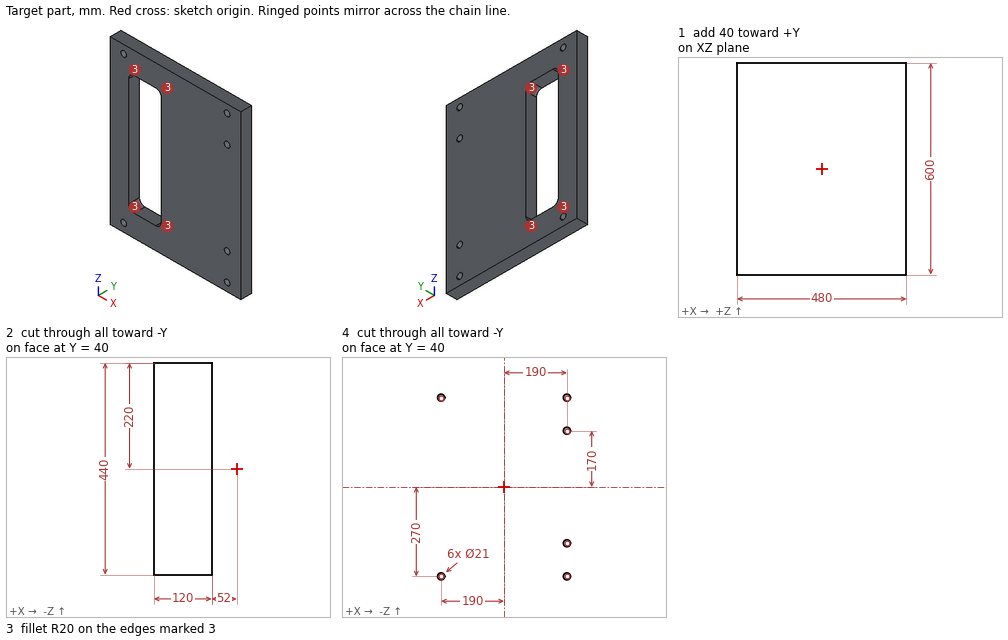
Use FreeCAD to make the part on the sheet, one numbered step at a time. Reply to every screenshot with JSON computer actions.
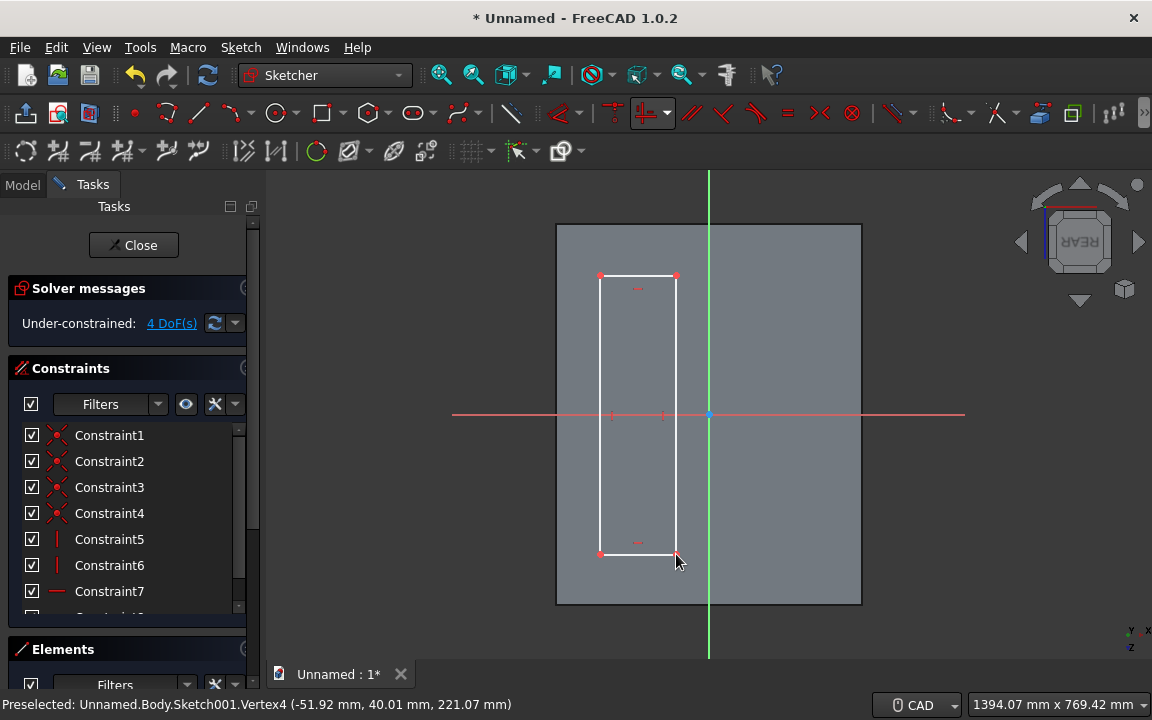
{"action": "left_click", "coordinate": [600, 360]}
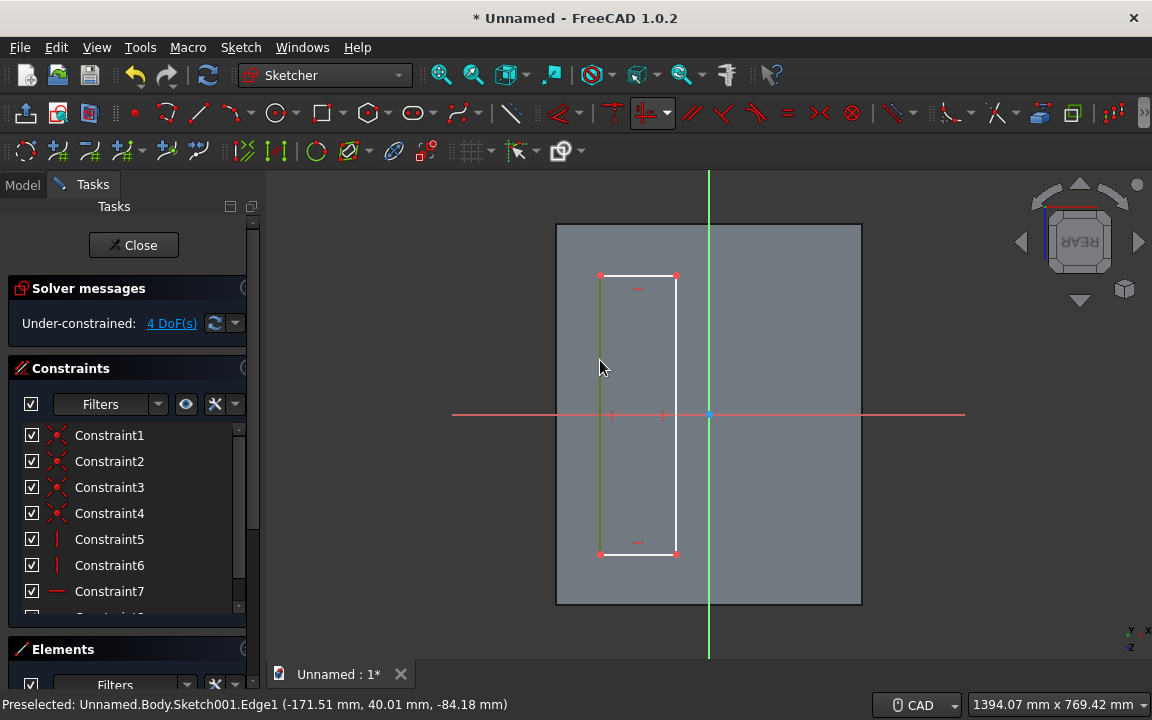
{"action": "left_click", "coordinate": [582, 114]}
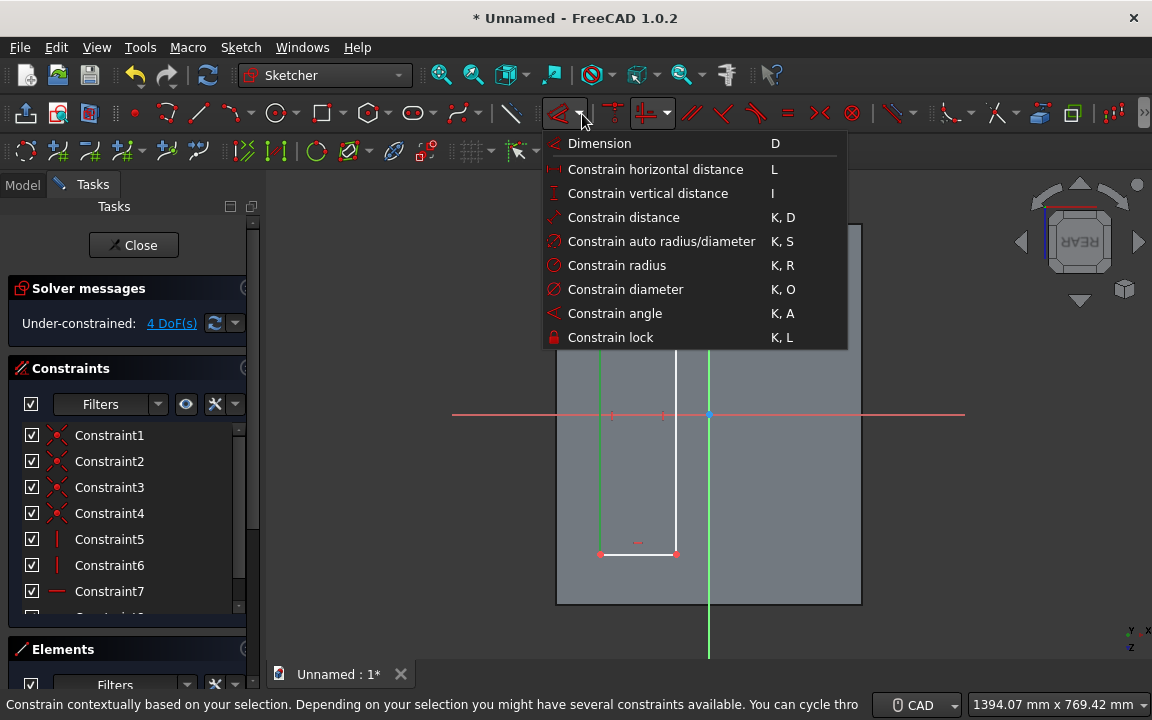
{"action": "left_click", "coordinate": [695, 193]}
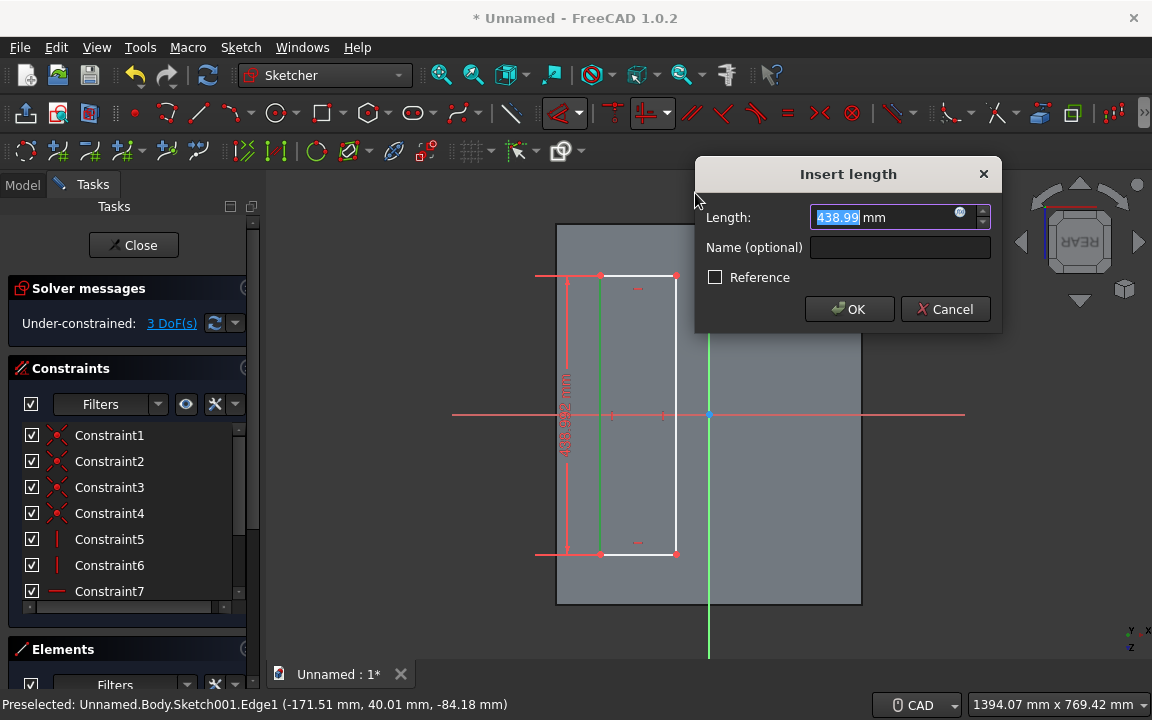
{"action": "type", "text": "440"}
{"action": "key", "text": "Return"}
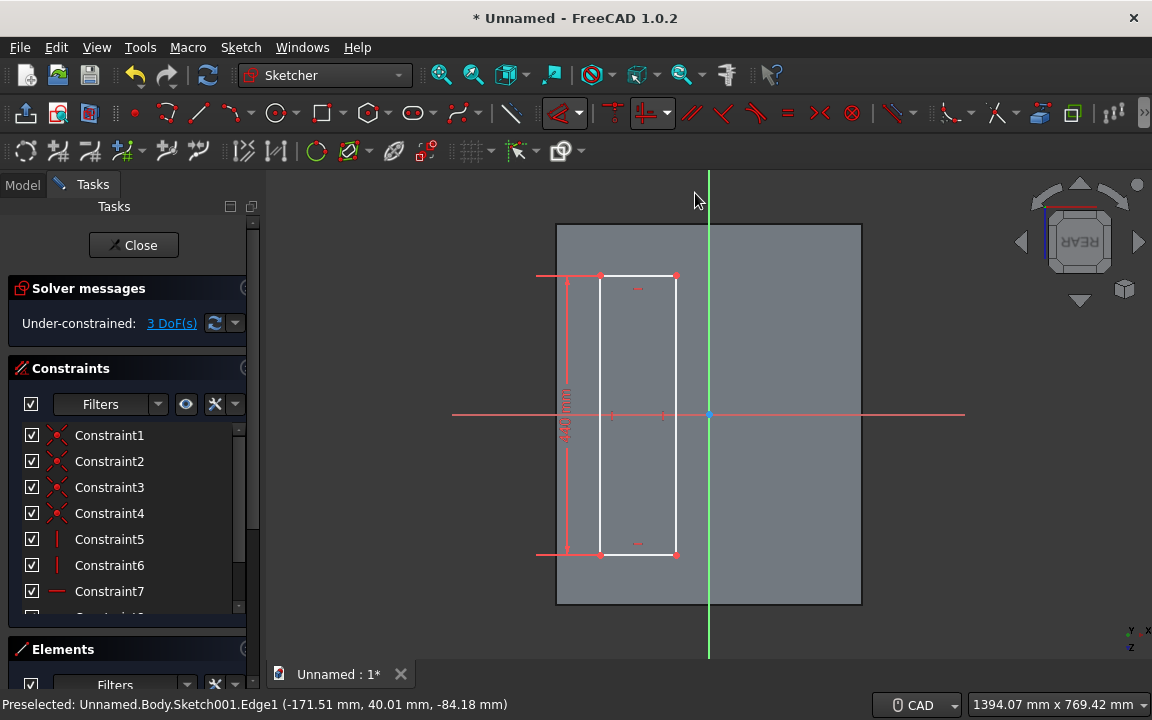
{"action": "left_click", "coordinate": [623, 555]}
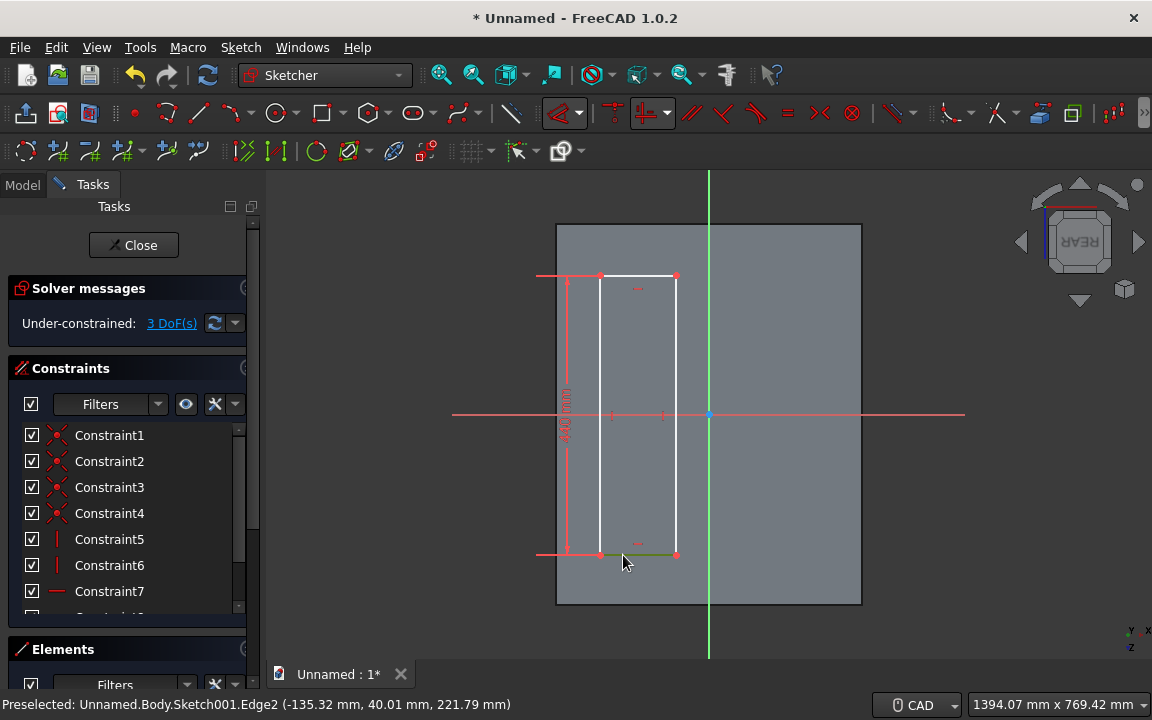
{"action": "key", "text": "l"}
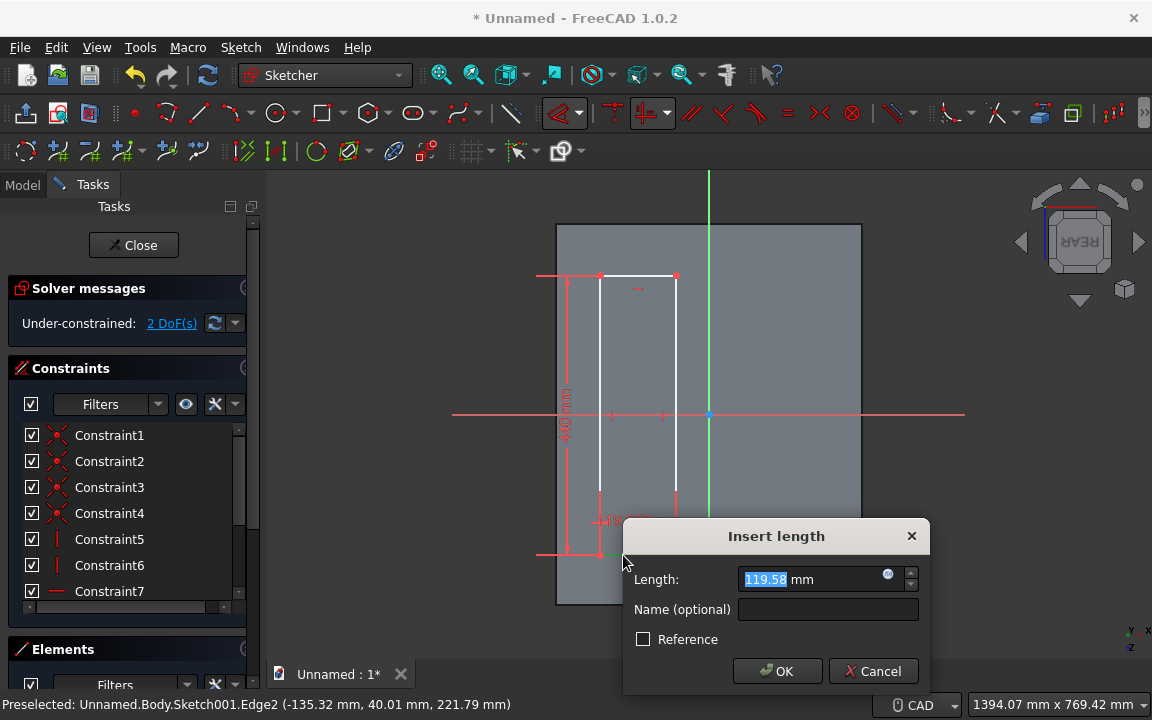
{"action": "type", "text": "120"}
{"action": "key", "text": "Return"}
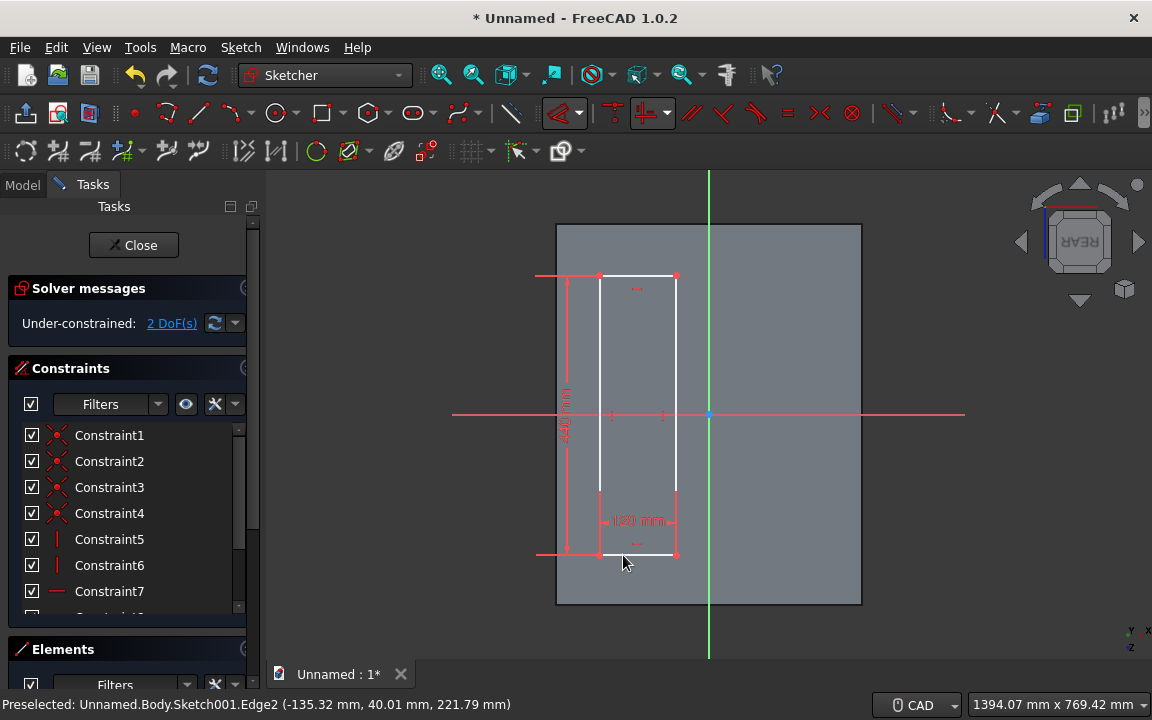
{"action": "left_click", "coordinate": [676, 555]}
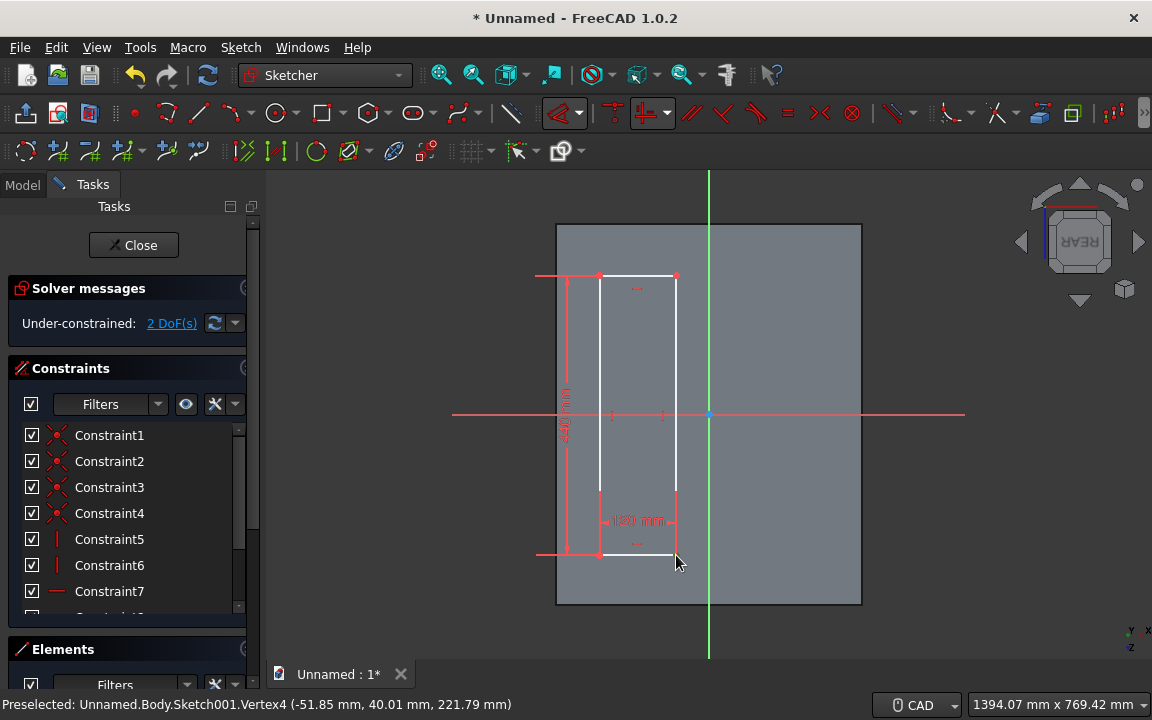
{"action": "left_click", "coordinate": [582, 114]}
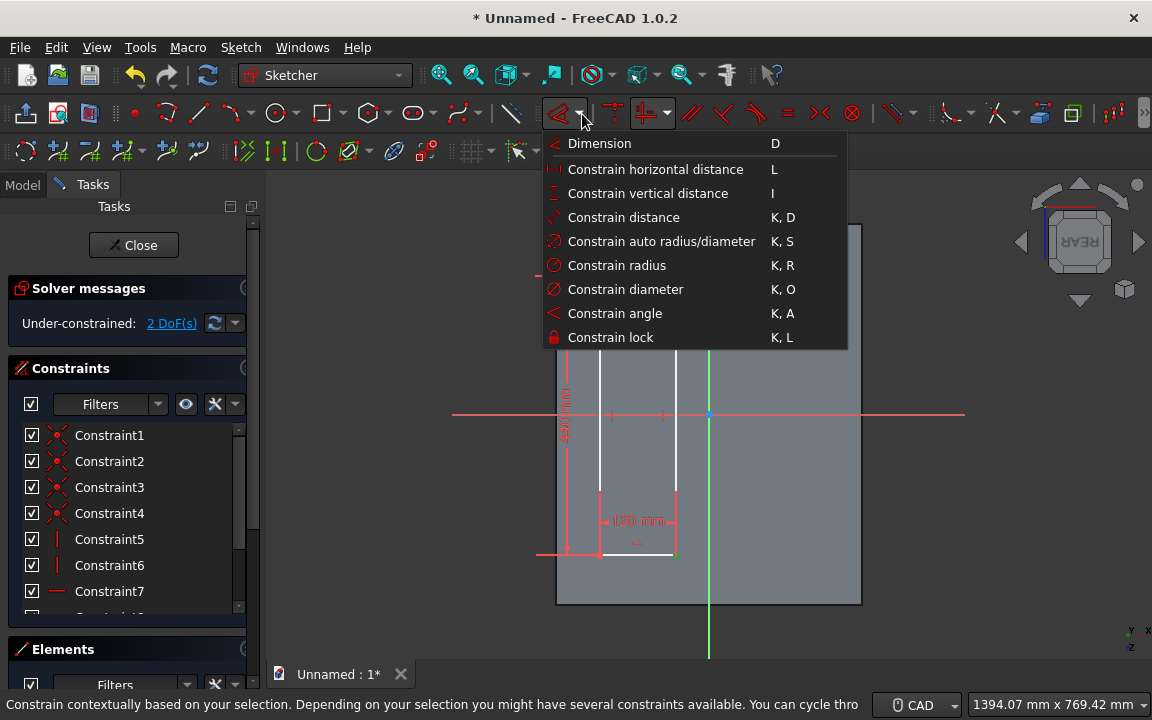
{"action": "left_click", "coordinate": [695, 169]}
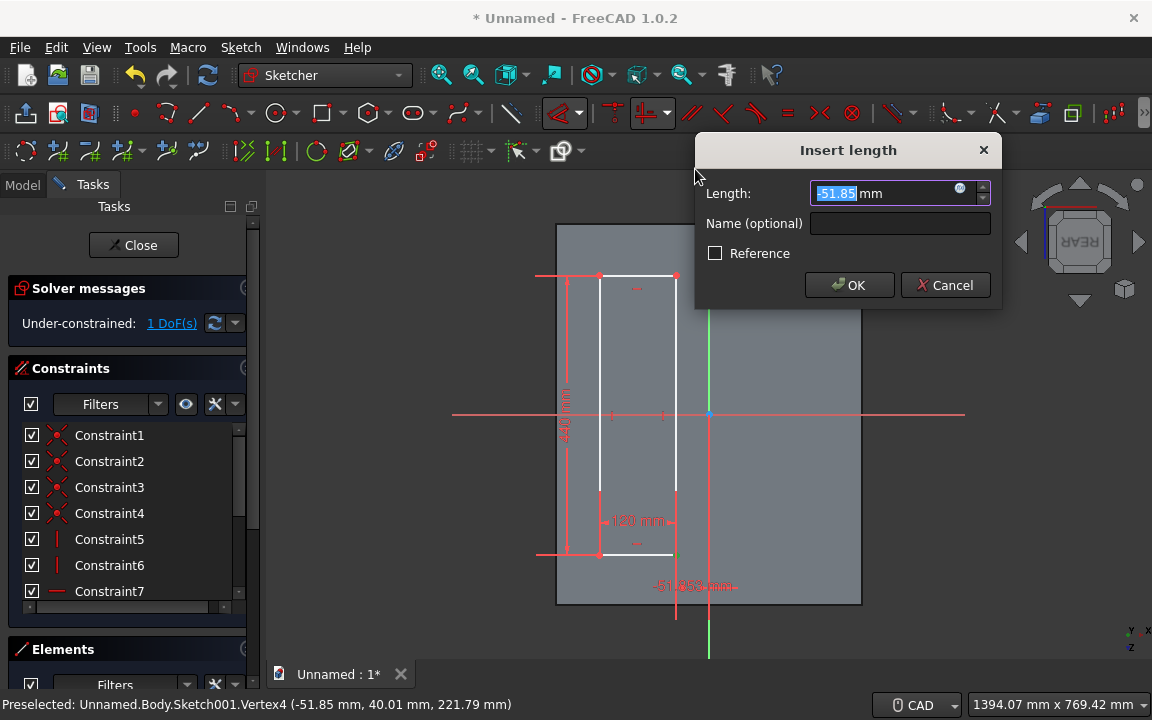
{"action": "type", "text": "-52"}
{"action": "key", "text": "Return"}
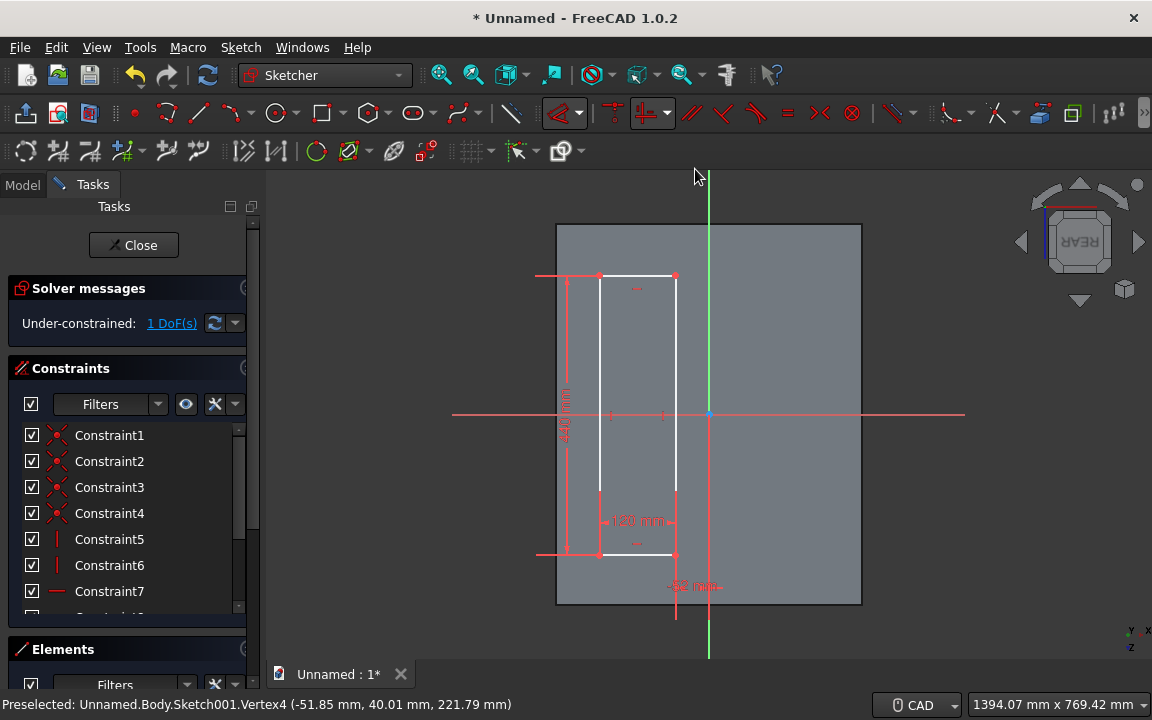
{"action": "left_click", "coordinate": [600, 276]}